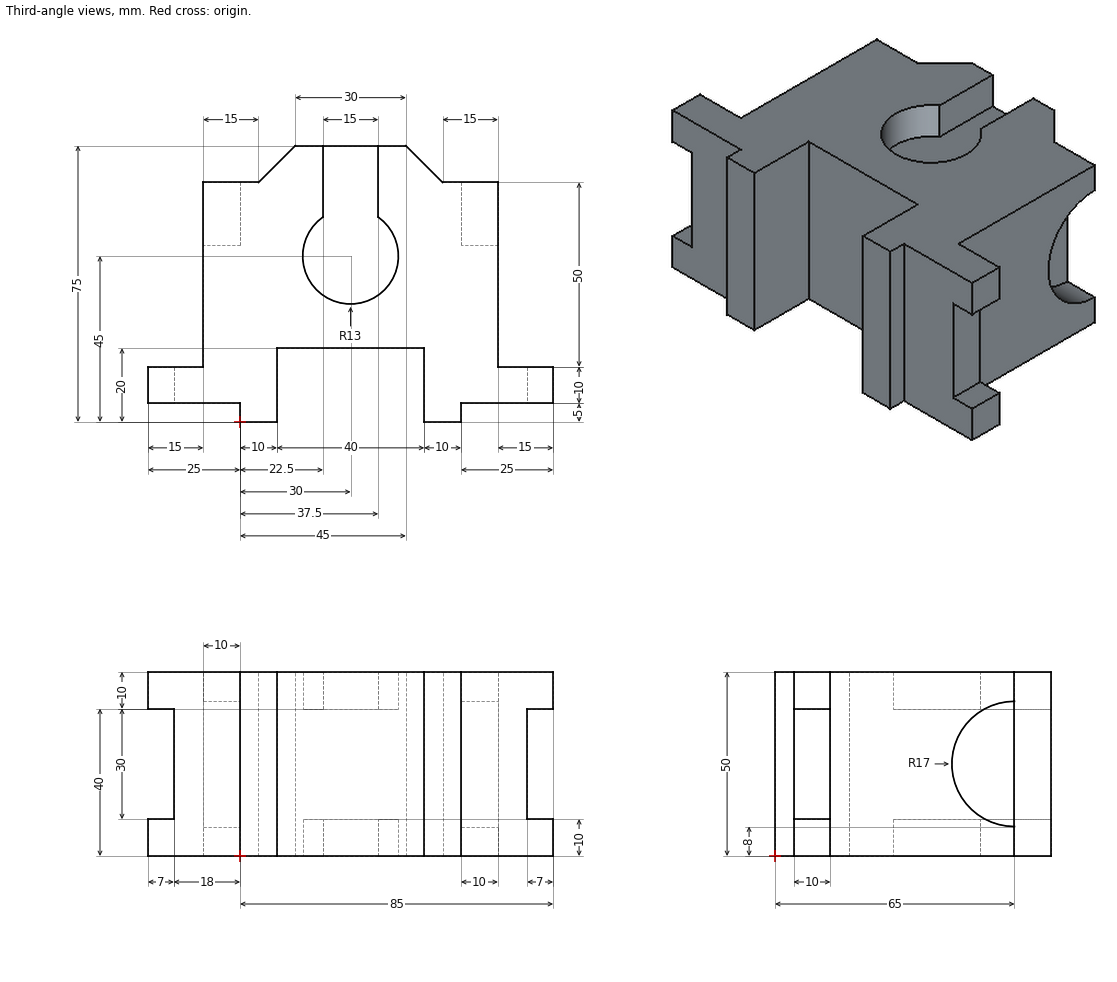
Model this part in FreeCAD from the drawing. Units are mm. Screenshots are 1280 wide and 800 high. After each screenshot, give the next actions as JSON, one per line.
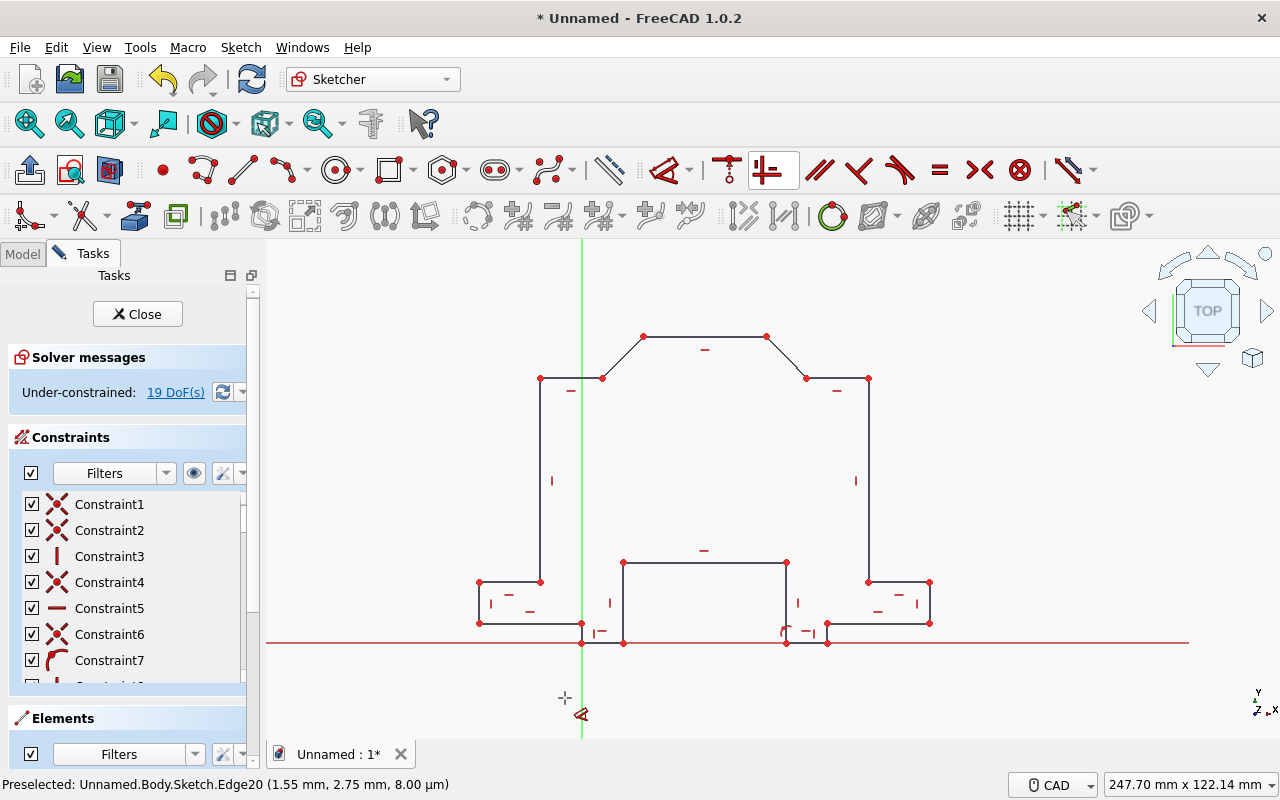
{"action": "scroll", "coordinate": [827, 637], "scroll_direction": "up", "scroll_amount": 5}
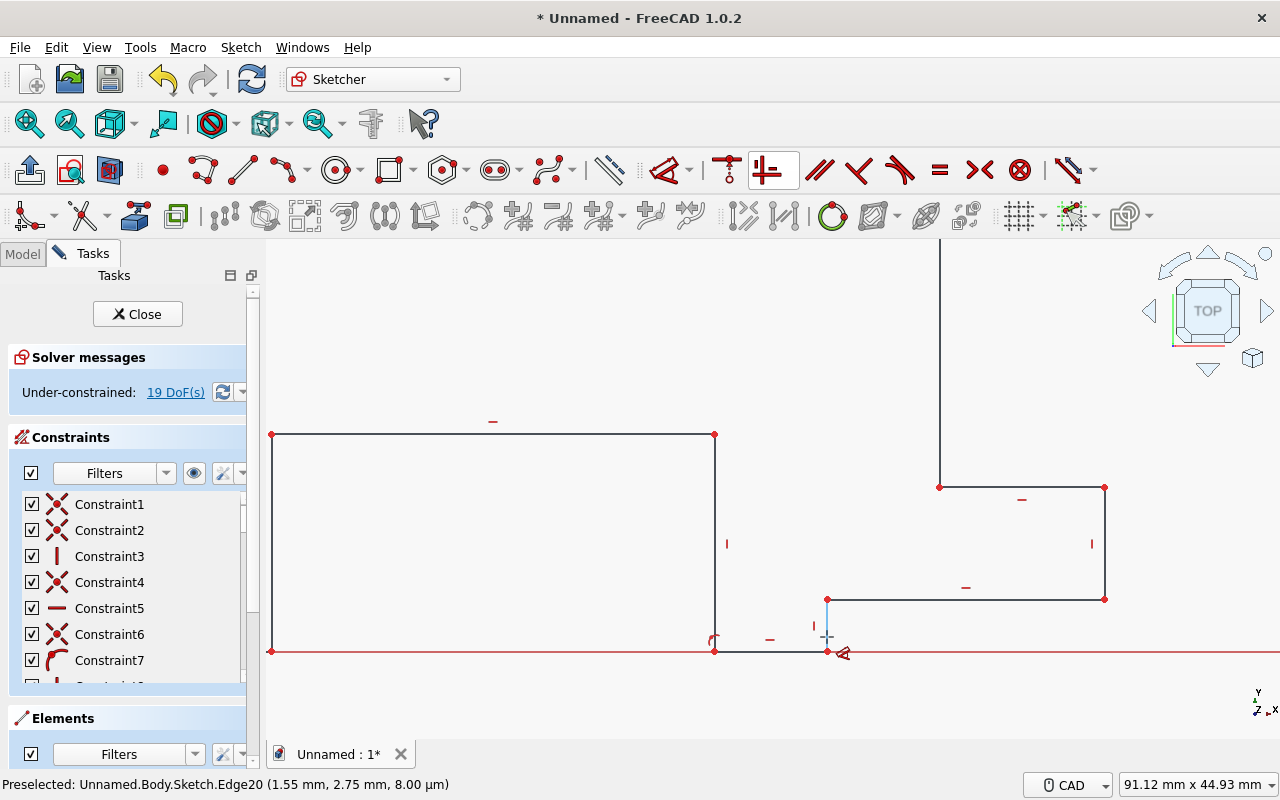
{"action": "left_click", "coordinate": [827, 636]}
{"action": "left_click", "coordinate": [861, 626]}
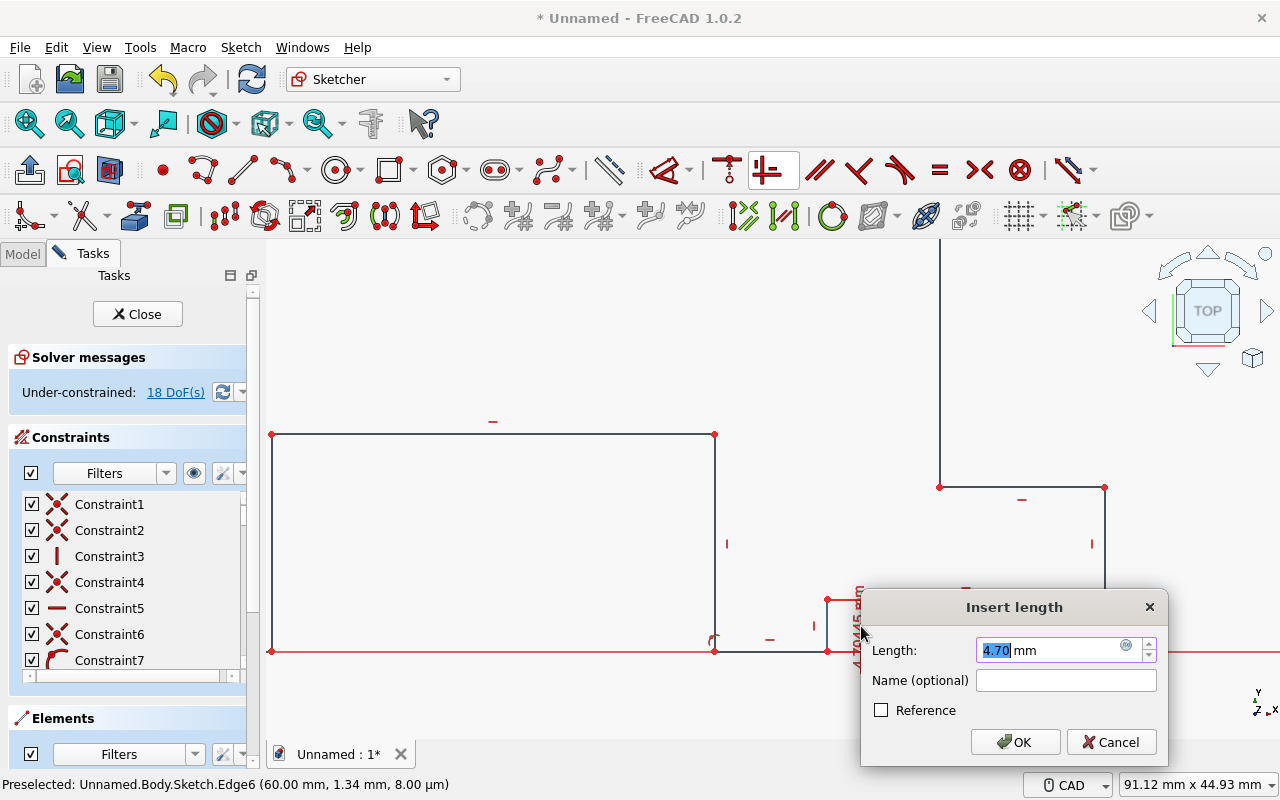
{"action": "type", "text": "5"}
{"action": "key", "text": "Return"}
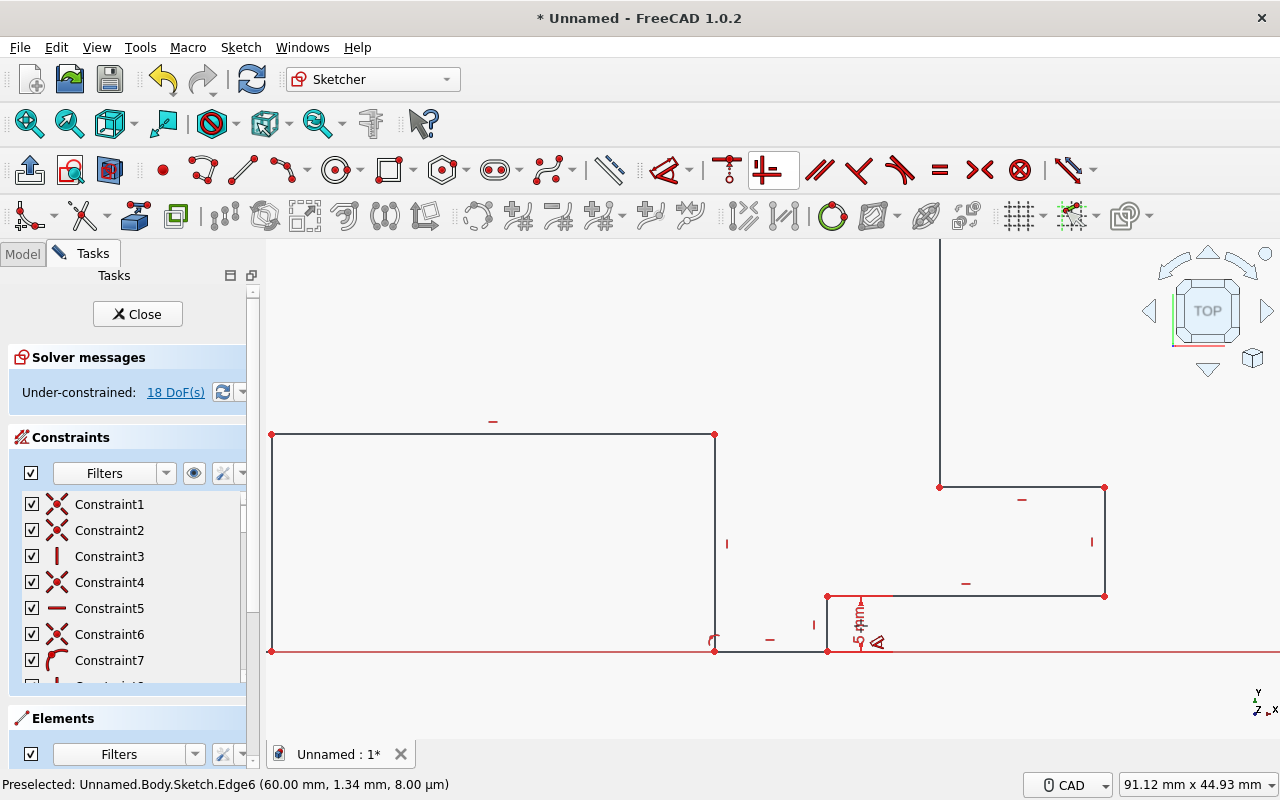
{"action": "scroll", "coordinate": [827, 637], "scroll_direction": "down", "scroll_amount": 5}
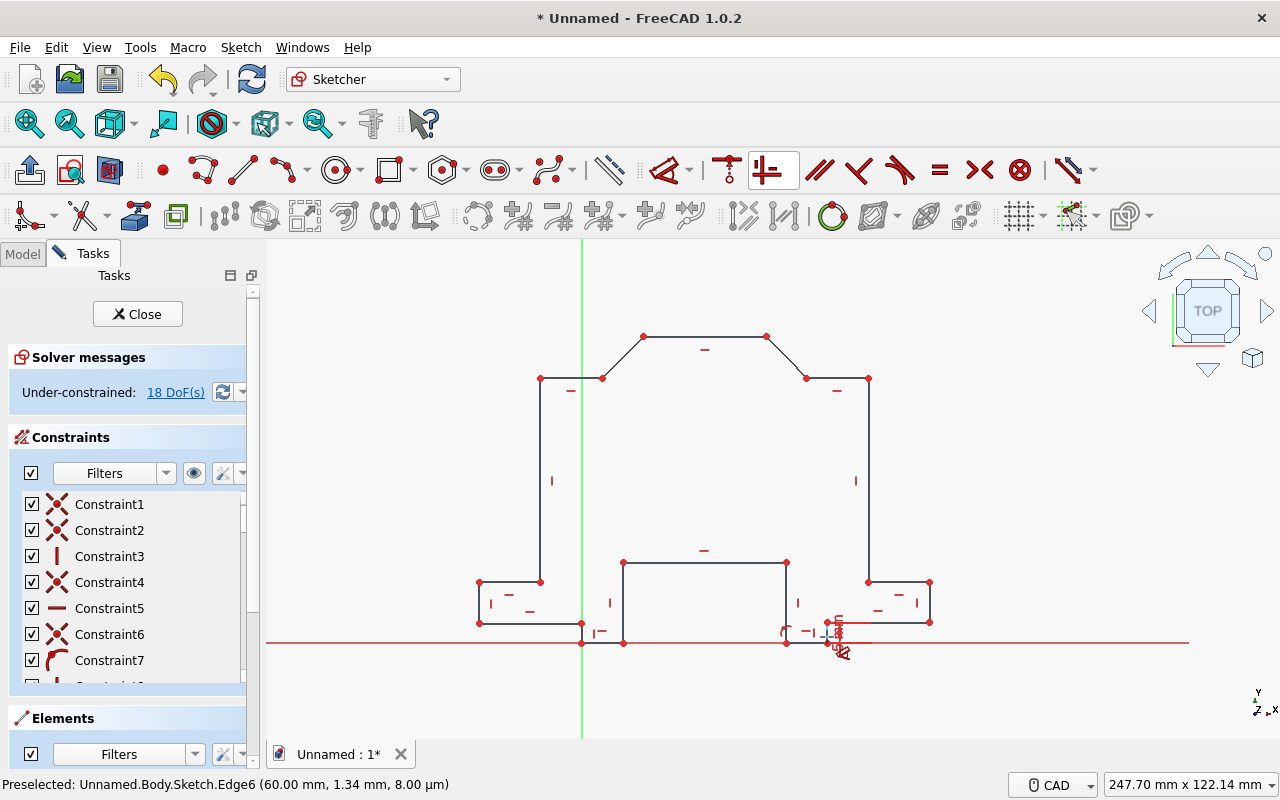
{"action": "scroll", "coordinate": [582, 630], "scroll_direction": "up", "scroll_amount": 5}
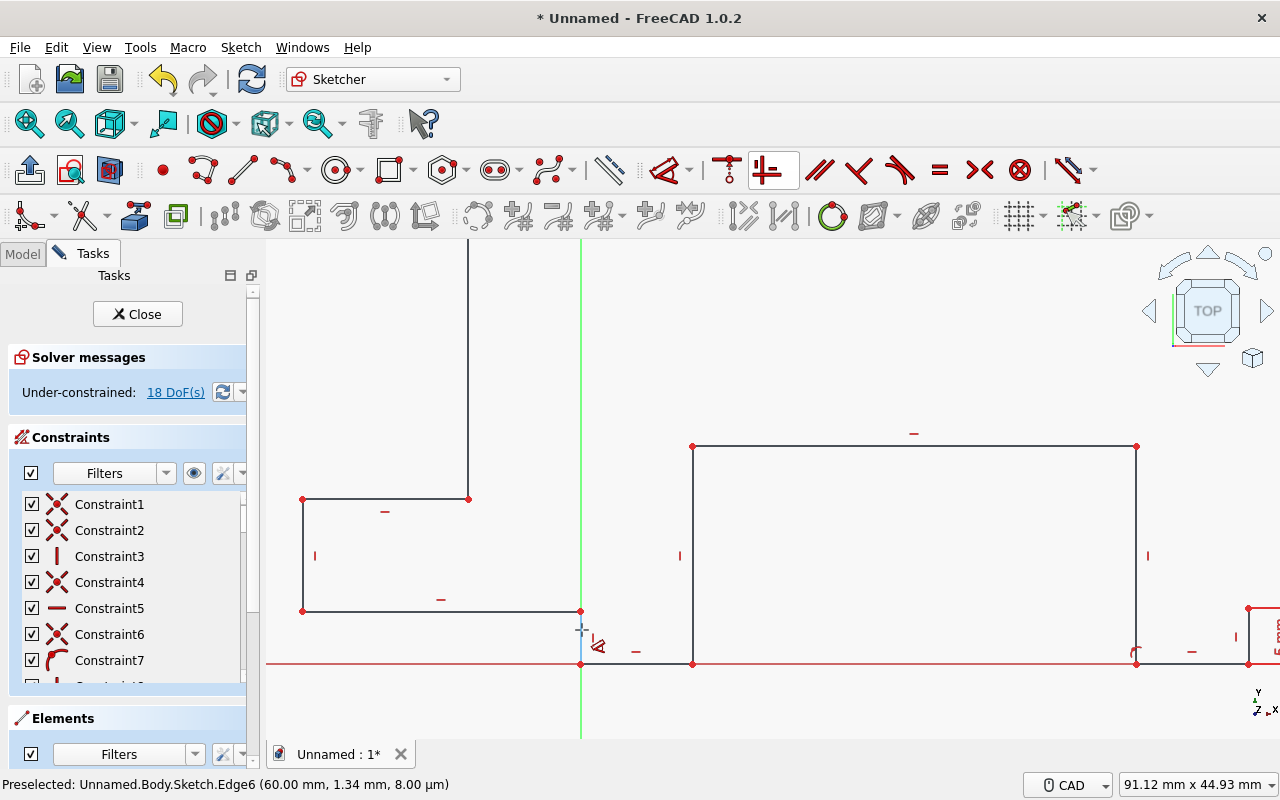
{"action": "left_click", "coordinate": [581, 627]}
{"action": "left_click", "coordinate": [547, 638]}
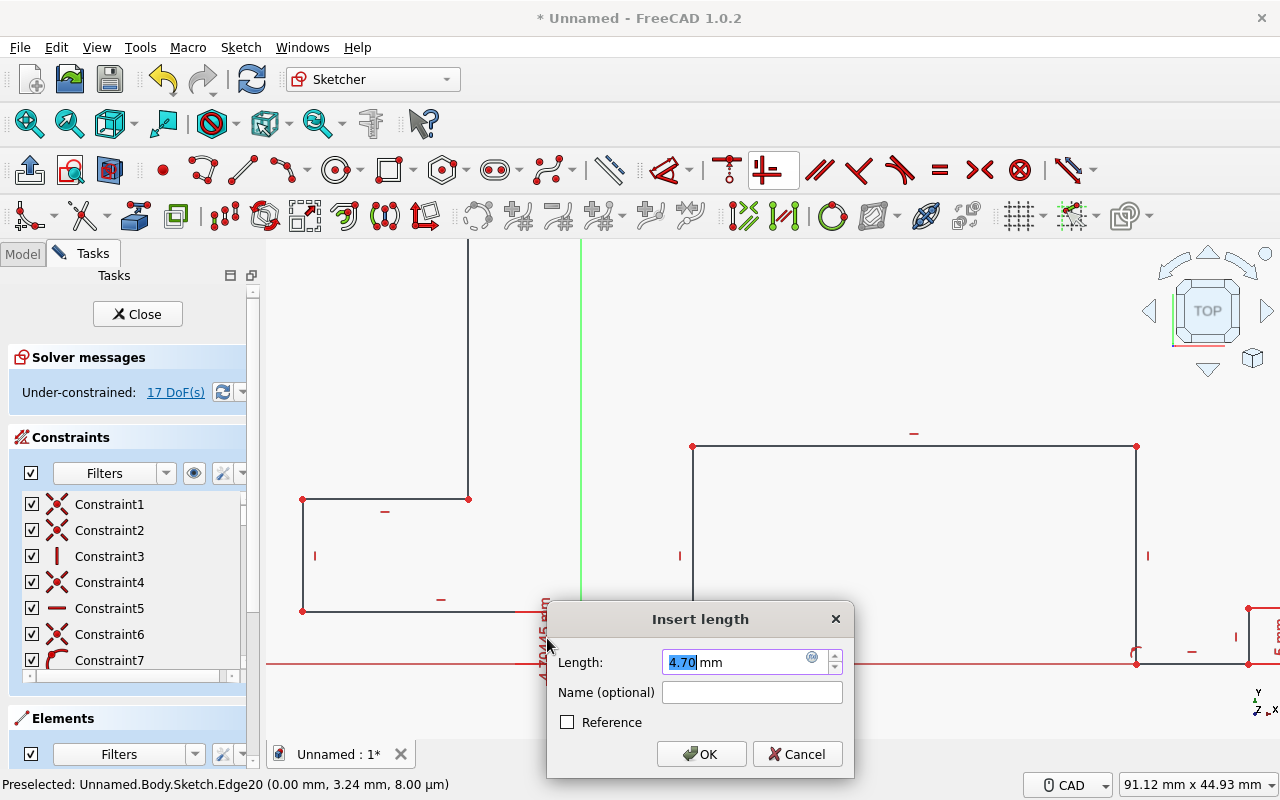
{"action": "type", "text": "5"}
{"action": "key", "text": "Return"}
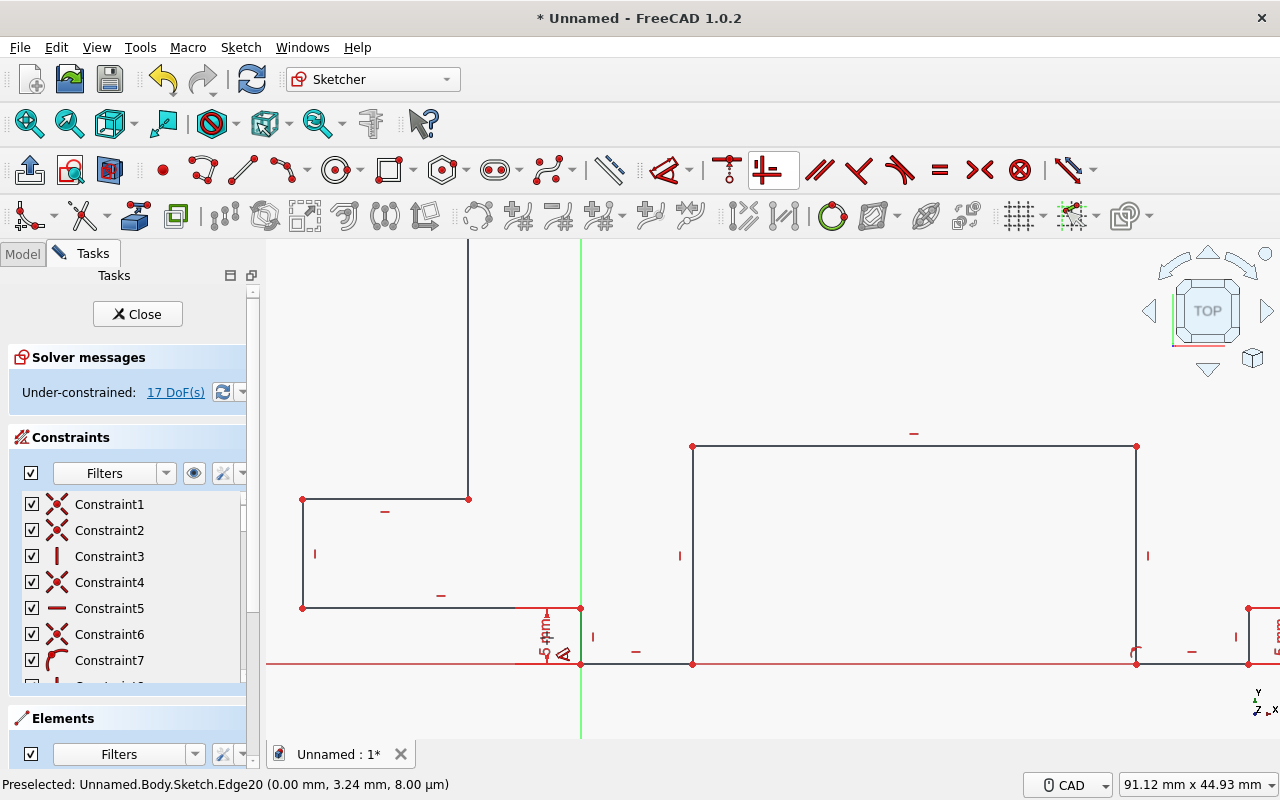
{"action": "left_click", "coordinate": [614, 664]}
{"action": "left_click", "coordinate": [637, 698]}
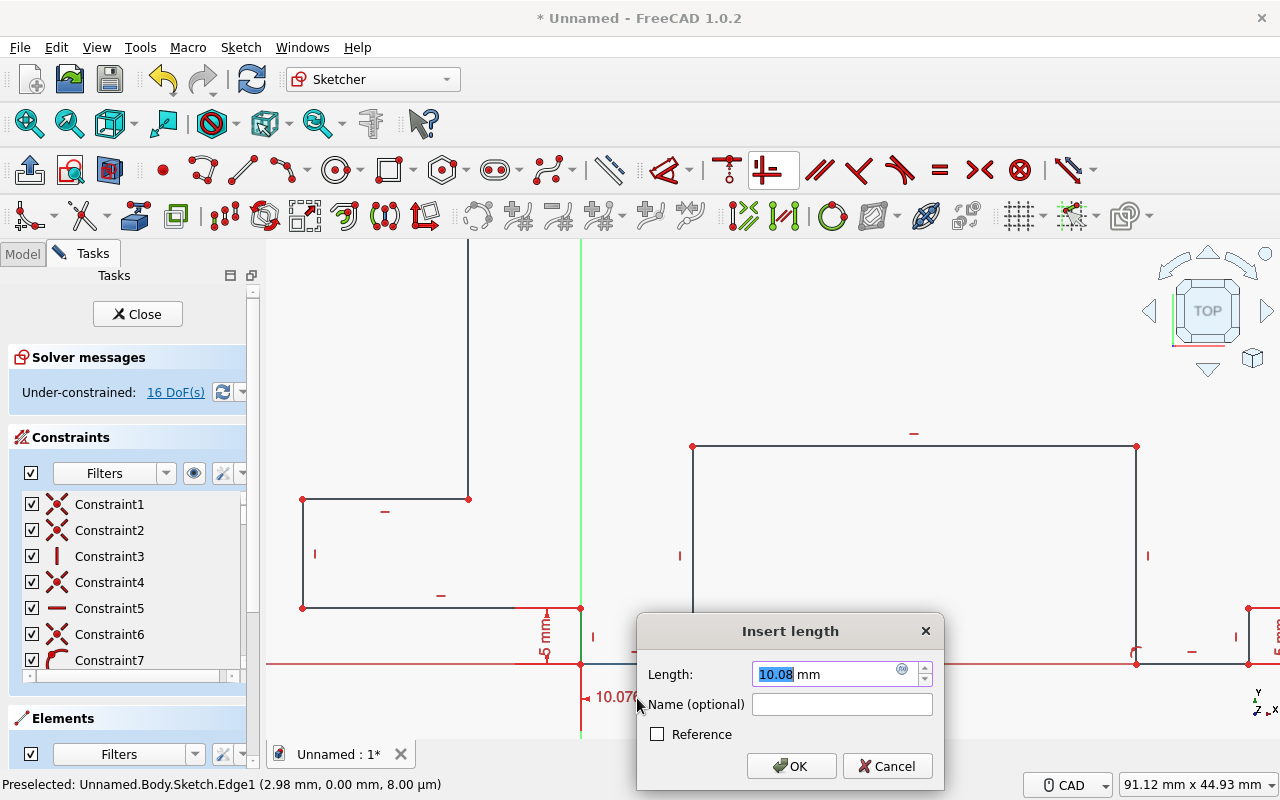
{"action": "type", "text": "10"}
{"action": "key", "text": "Return"}